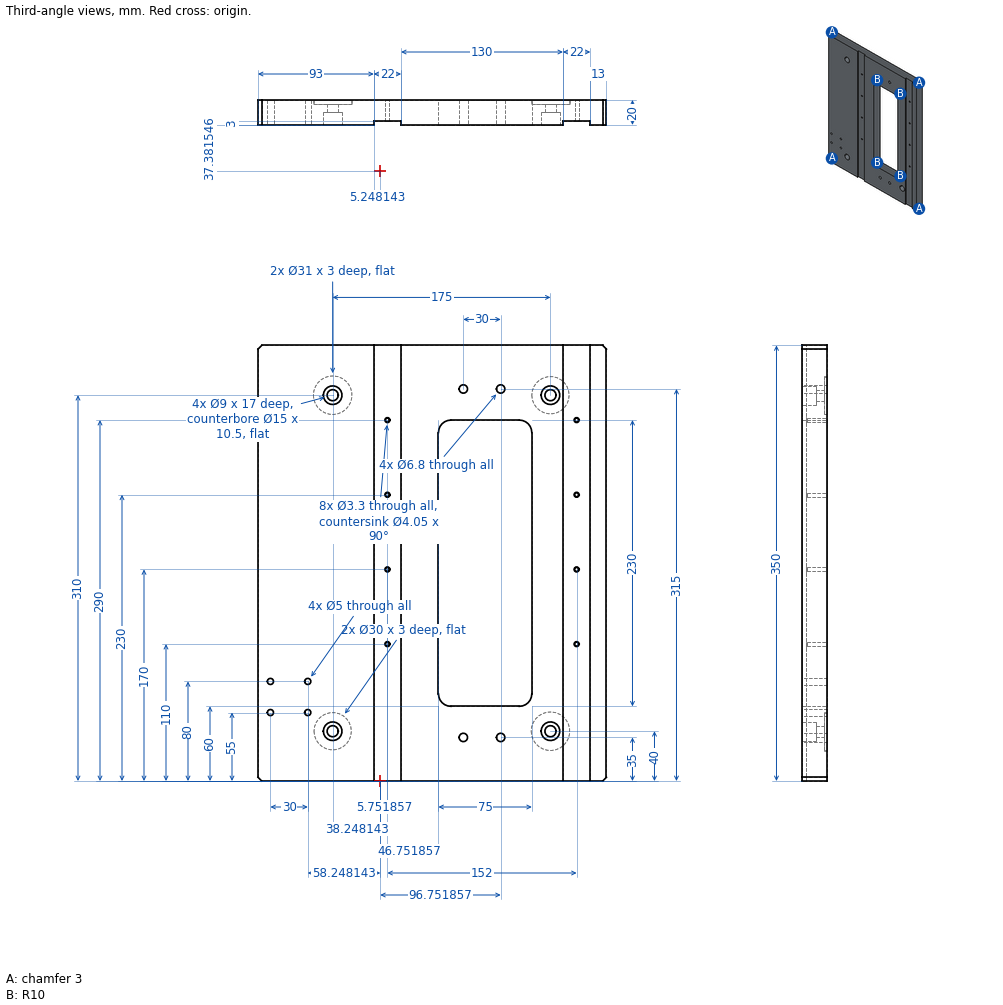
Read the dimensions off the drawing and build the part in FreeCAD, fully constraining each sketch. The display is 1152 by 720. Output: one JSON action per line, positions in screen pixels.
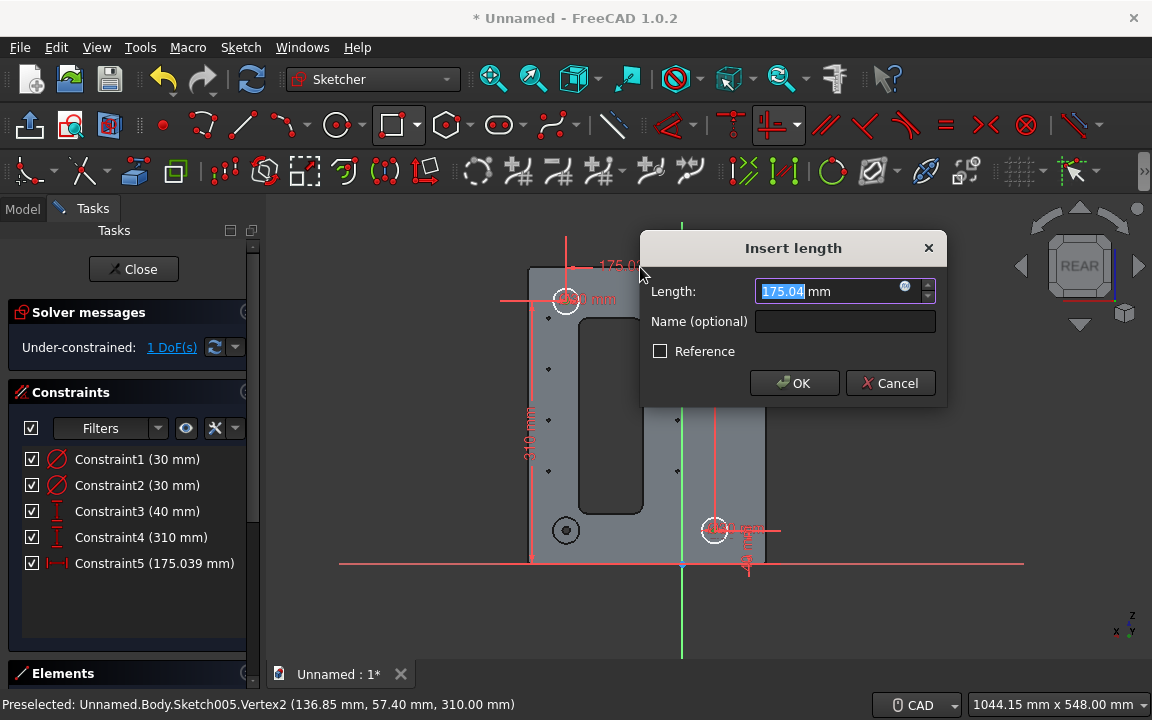
{"action": "type", "text": "175"}
{"action": "key", "text": "Return"}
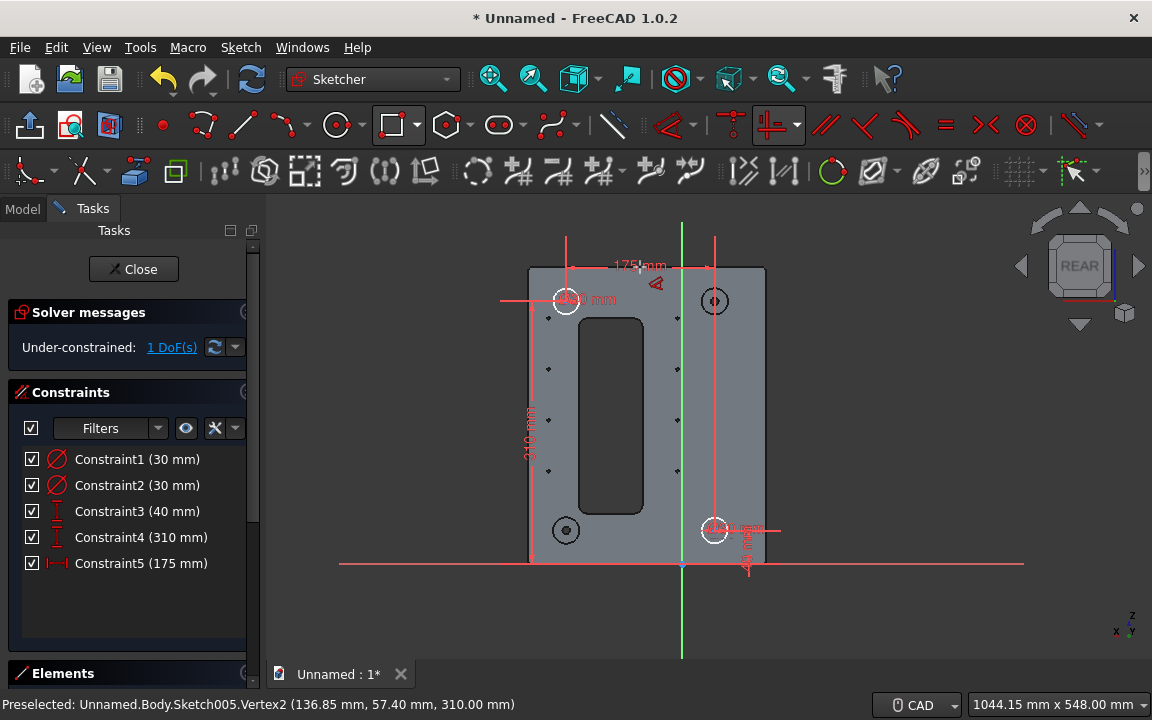
{"action": "scroll", "coordinate": [715, 531], "scroll_direction": "up", "scroll_amount": 2}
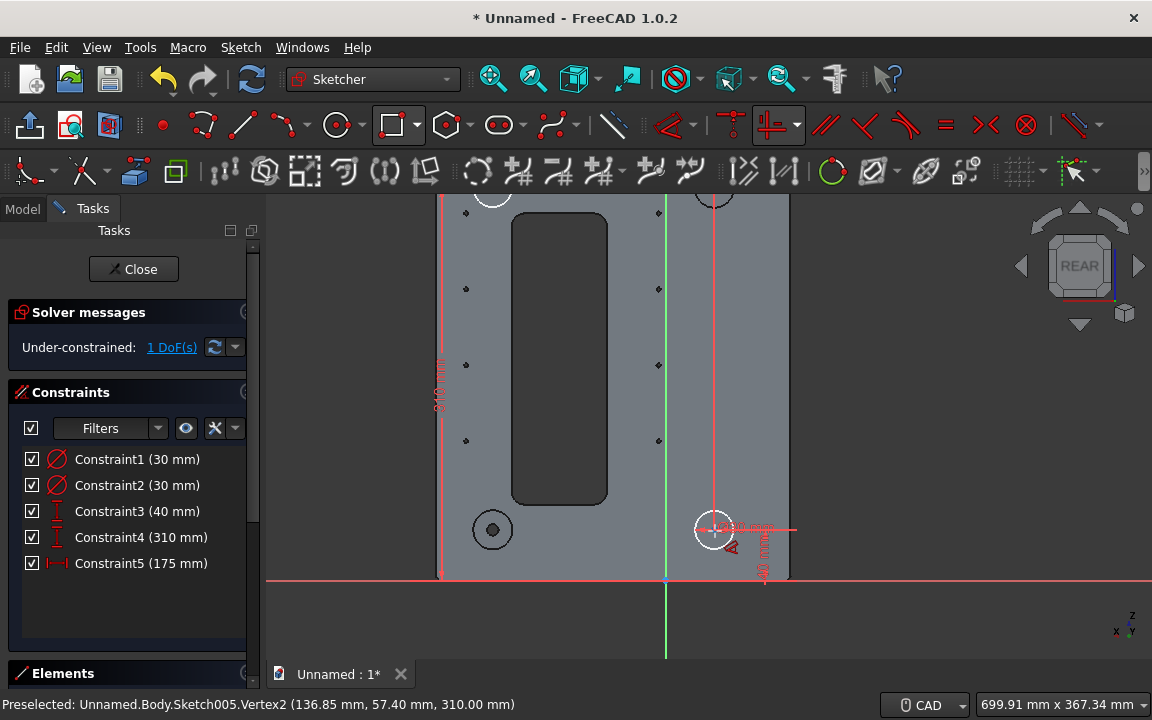
{"action": "left_click", "coordinate": [714, 530]}
{"action": "left_click", "coordinate": [690, 615]}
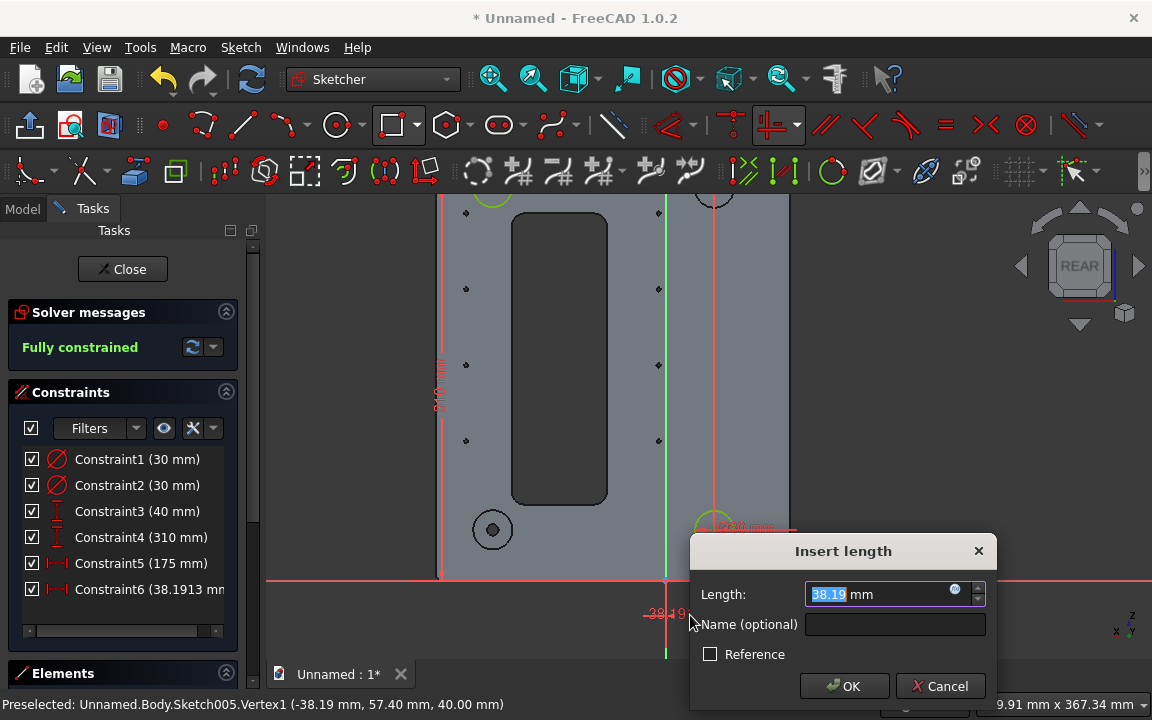
{"action": "type", "text": "38.248143"}
{"action": "key", "text": "Return"}
{"action": "key", "text": "Escape"}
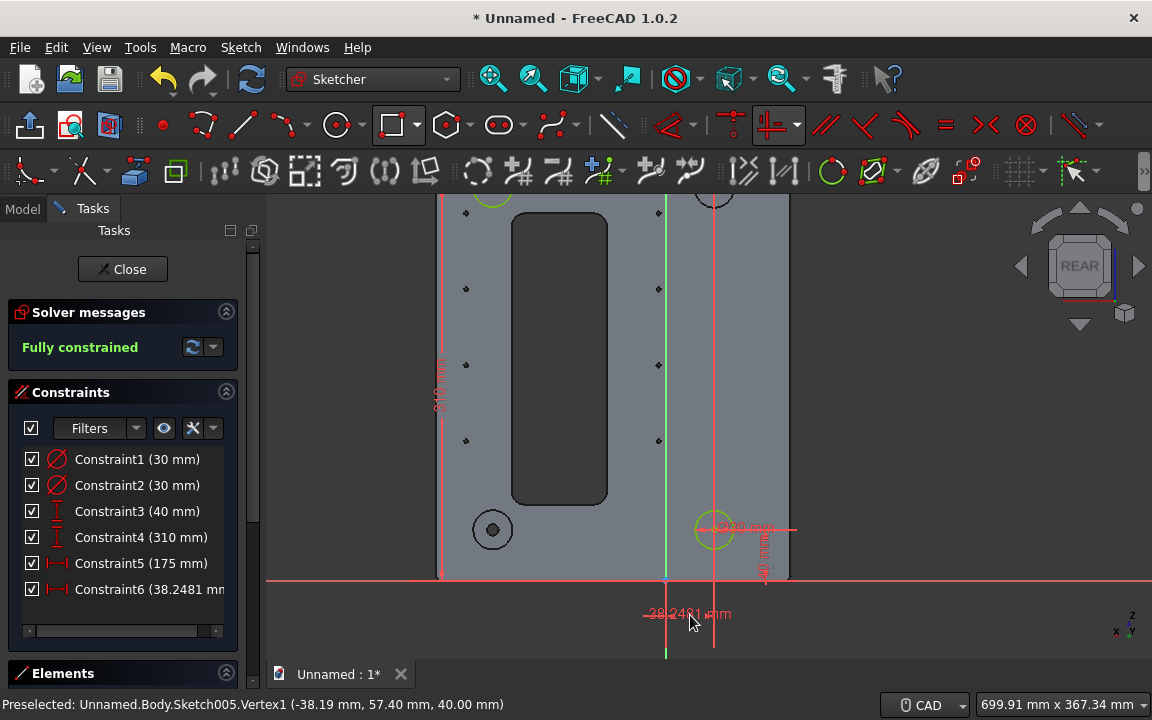
{"action": "left_click", "coordinate": [123, 269]}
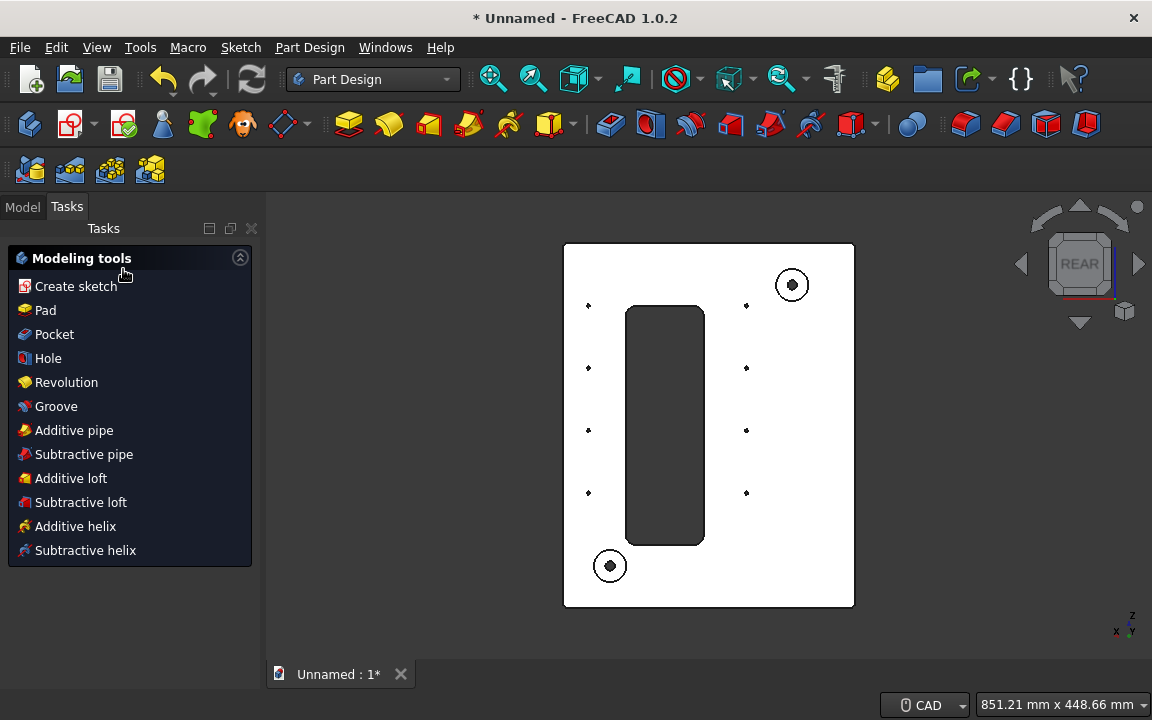
{"action": "left_click", "coordinate": [652, 124]}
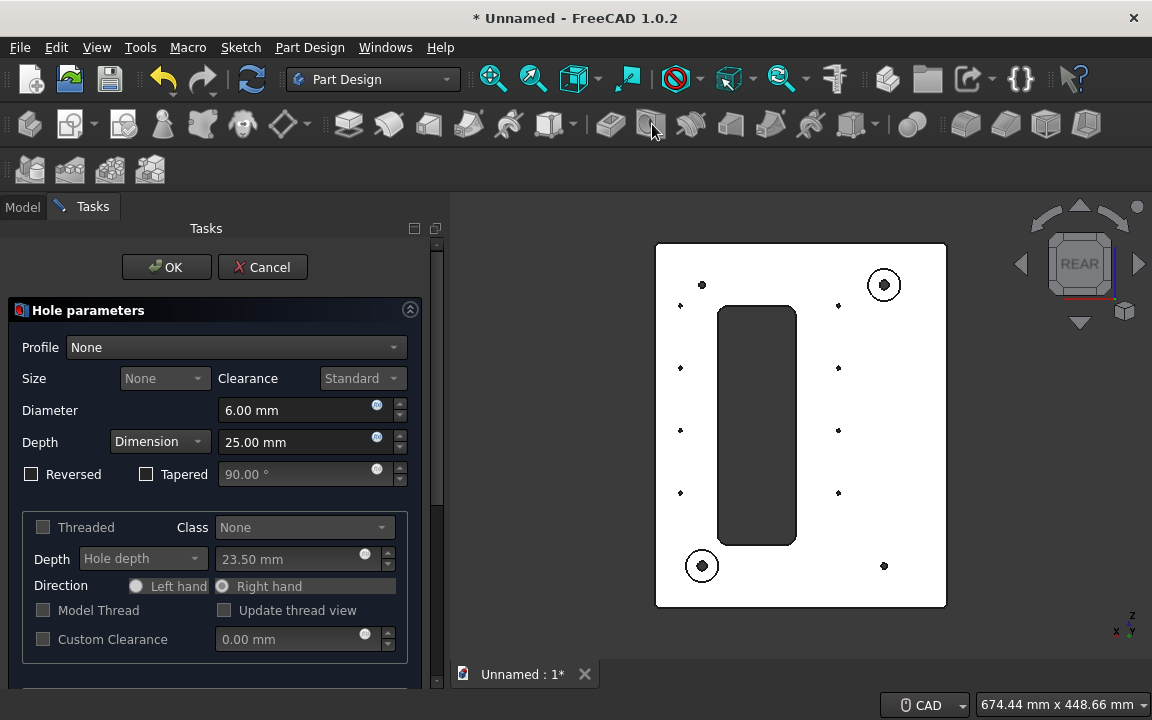
{"action": "triple_click", "coordinate": [305, 410]}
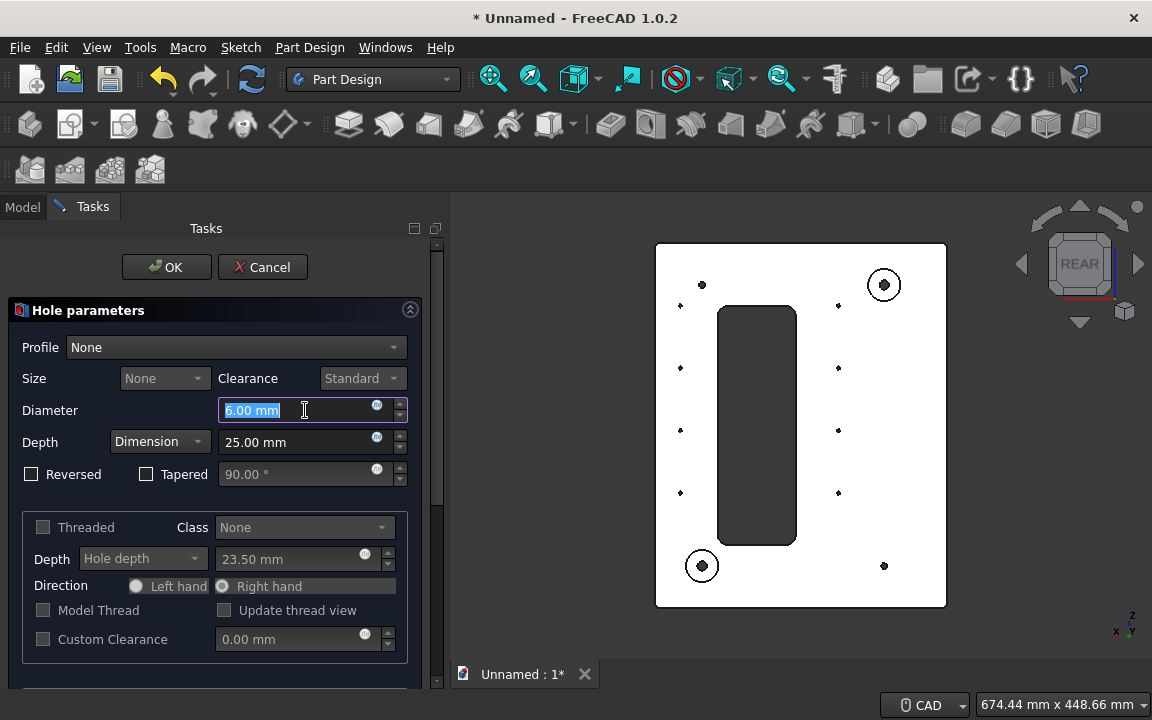
{"action": "type", "text": "30"}
{"action": "key", "text": "Tab"}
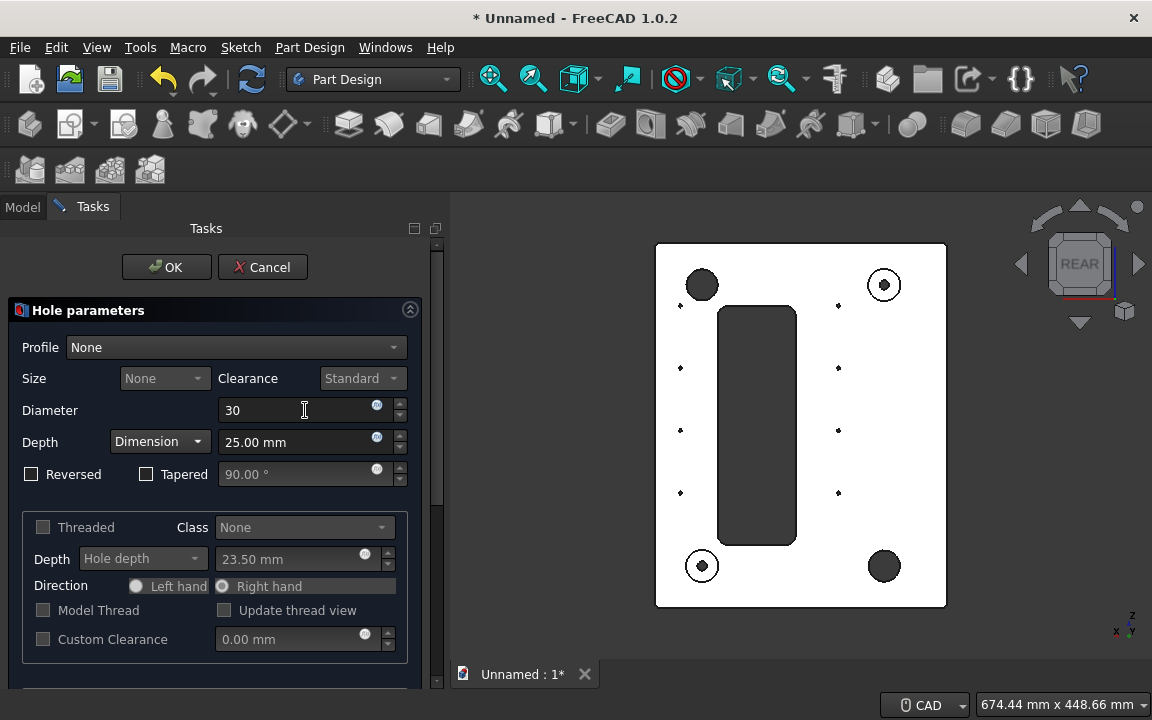
{"action": "triple_click", "coordinate": [305, 442]}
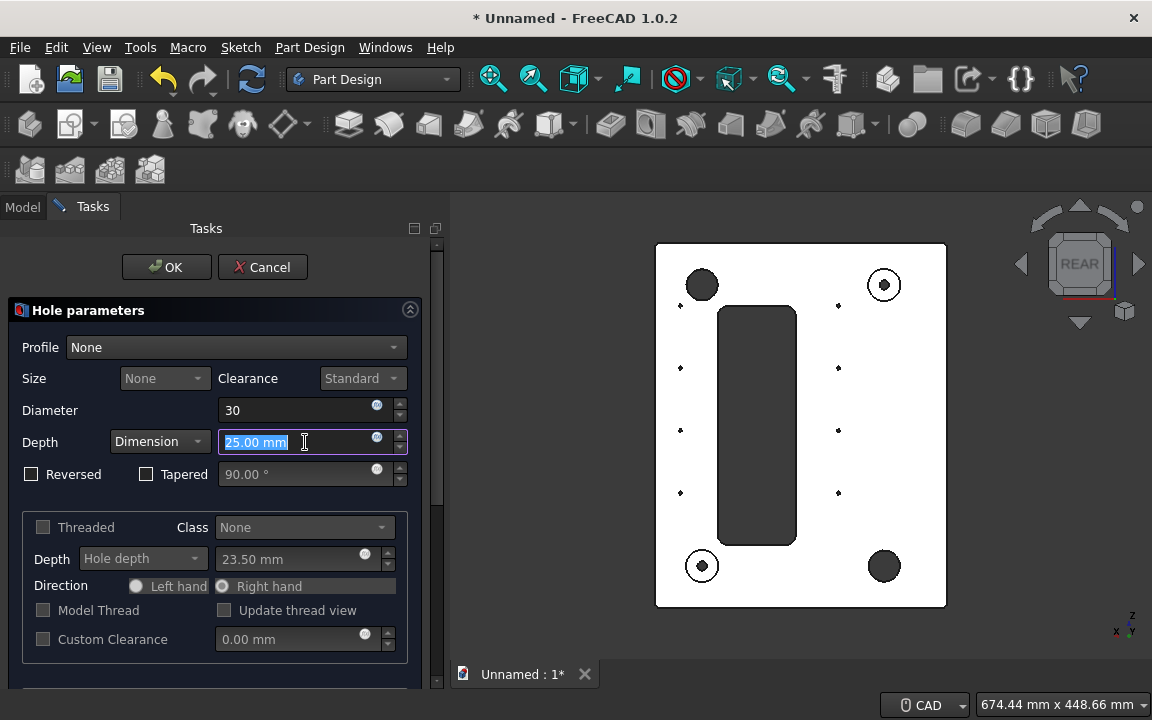
{"action": "type", "text": "3"}
{"action": "key", "text": "Tab"}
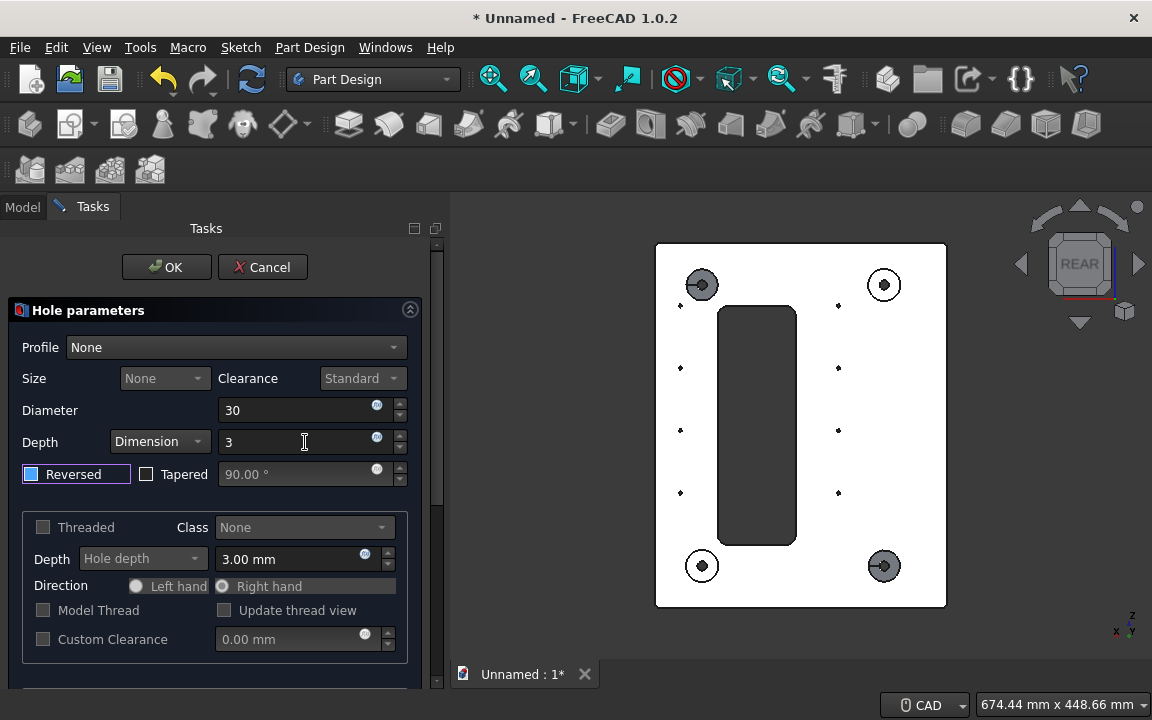
{"action": "scroll", "coordinate": [437, 463], "scroll_direction": "down", "scroll_amount": 5}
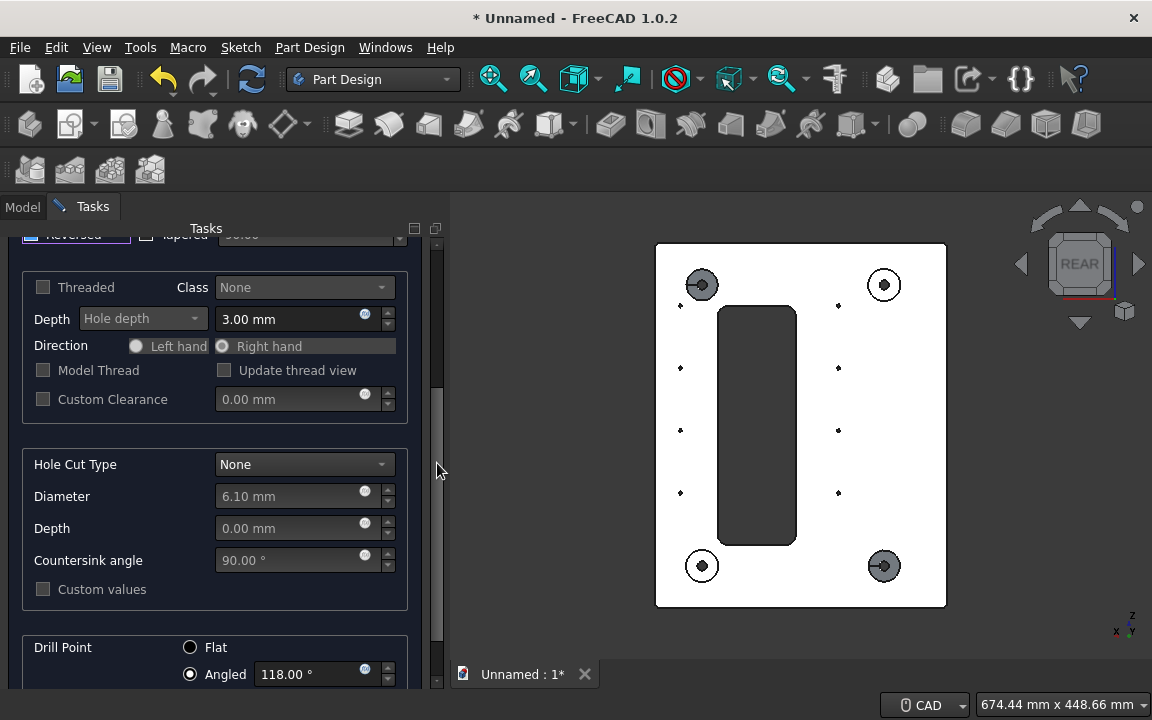
{"action": "left_click", "coordinate": [191, 589]}